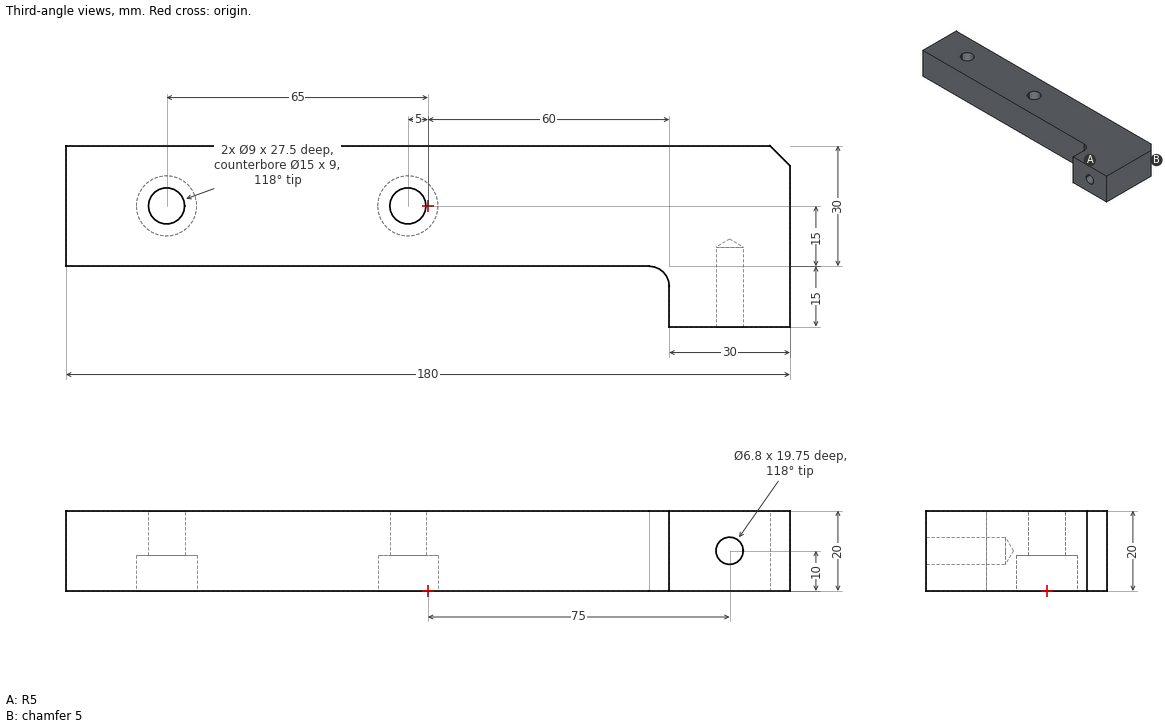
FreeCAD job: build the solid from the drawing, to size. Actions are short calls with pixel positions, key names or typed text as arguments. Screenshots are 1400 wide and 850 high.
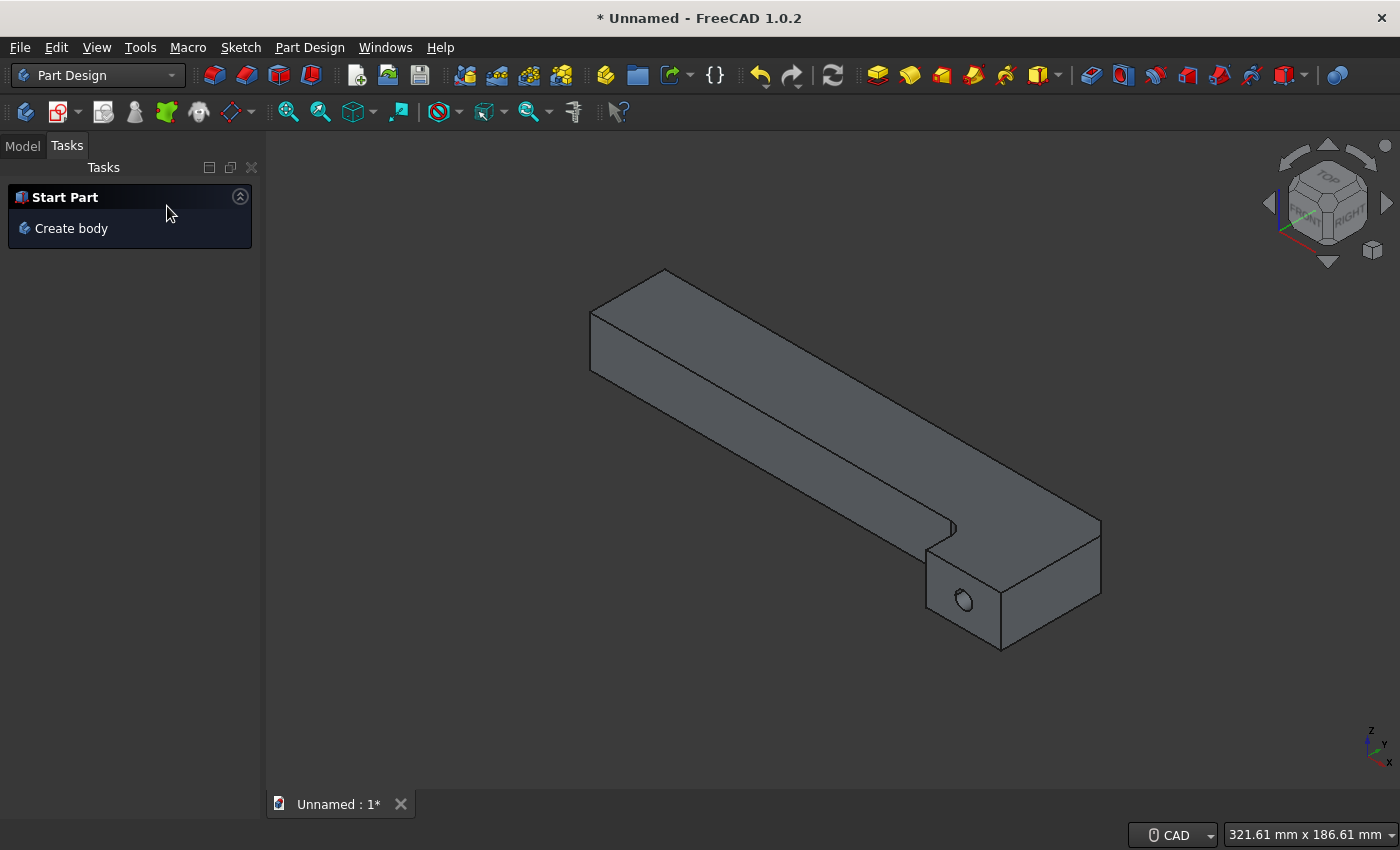
click(58, 112)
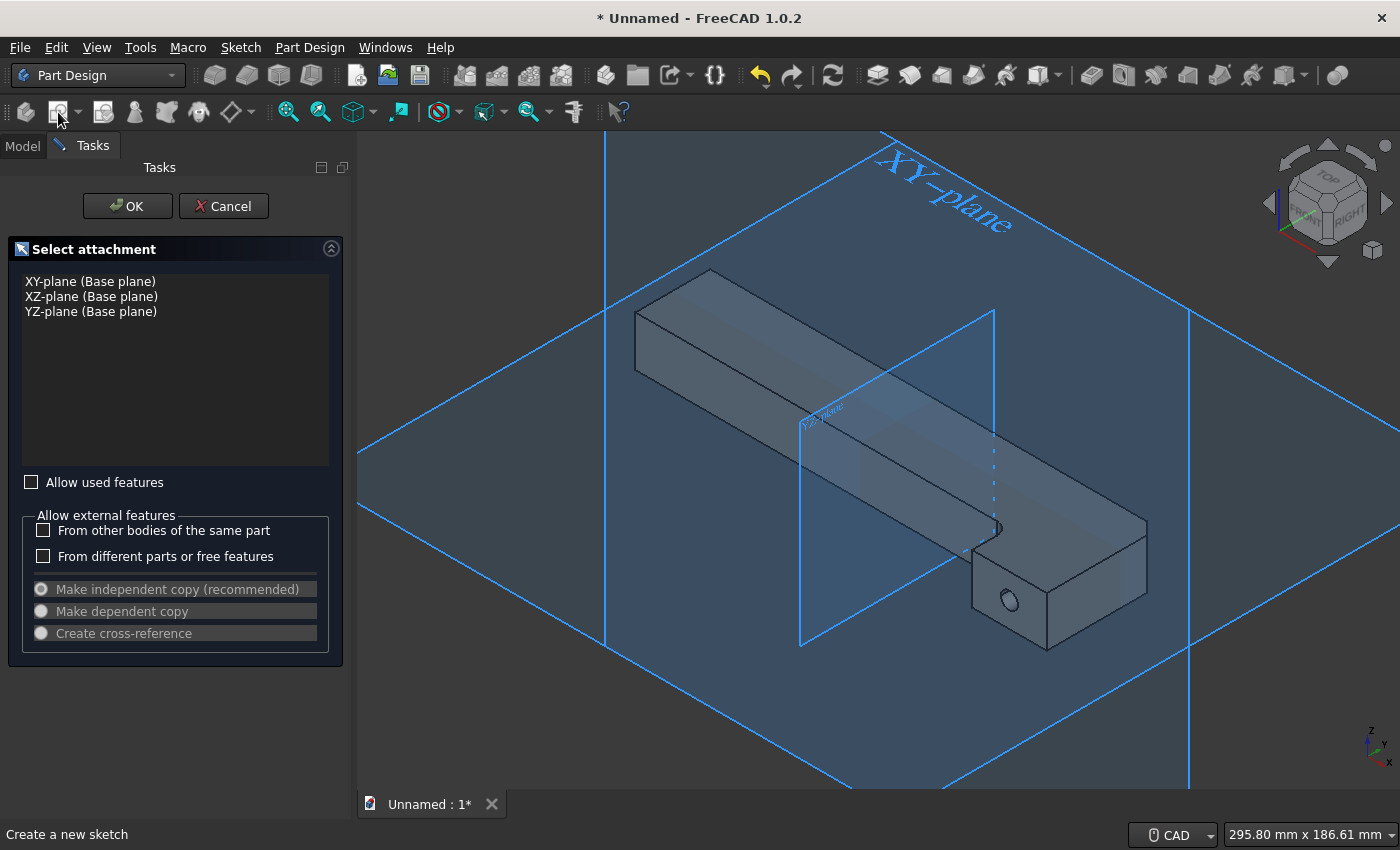
click(82, 282)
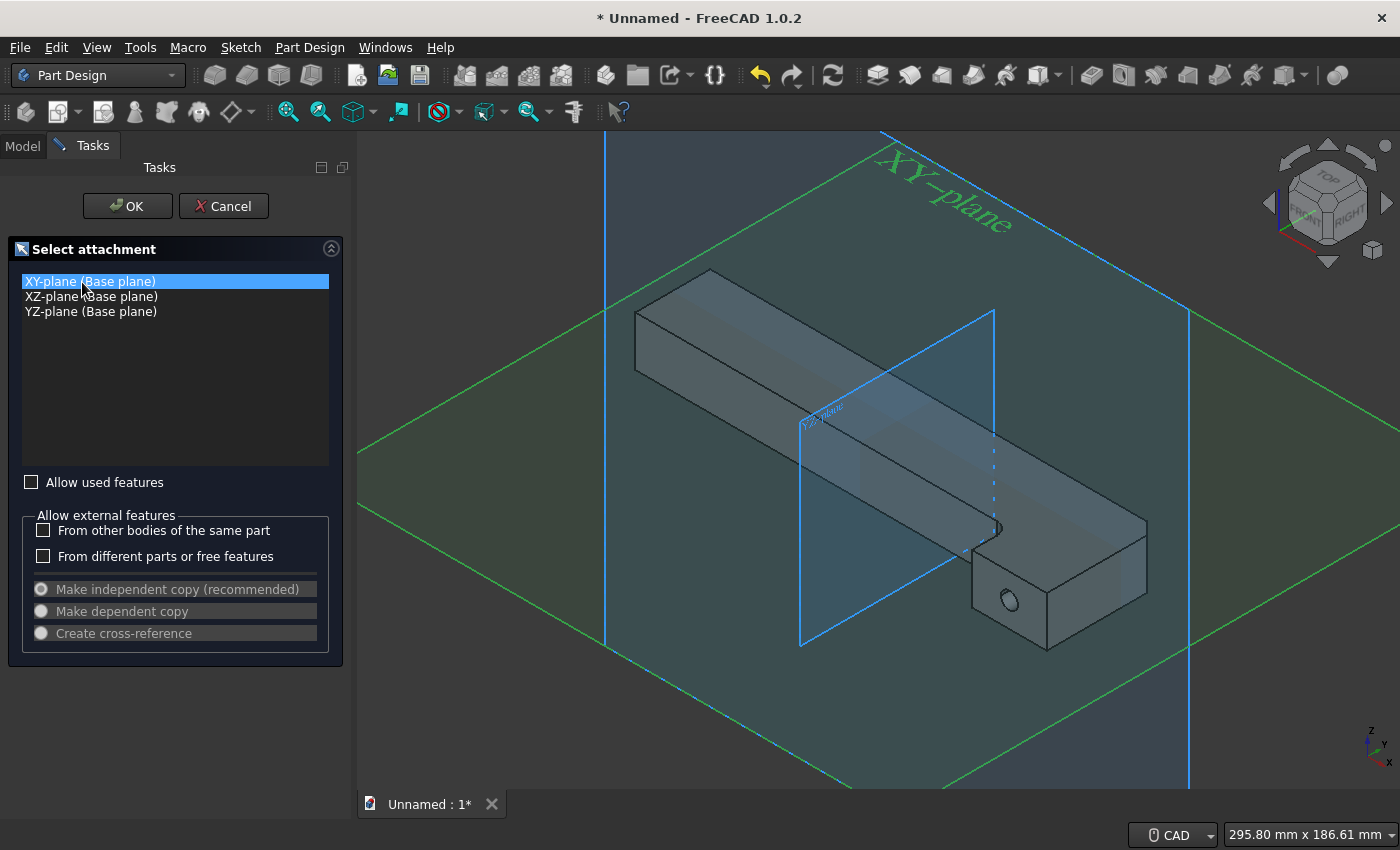
click(128, 206)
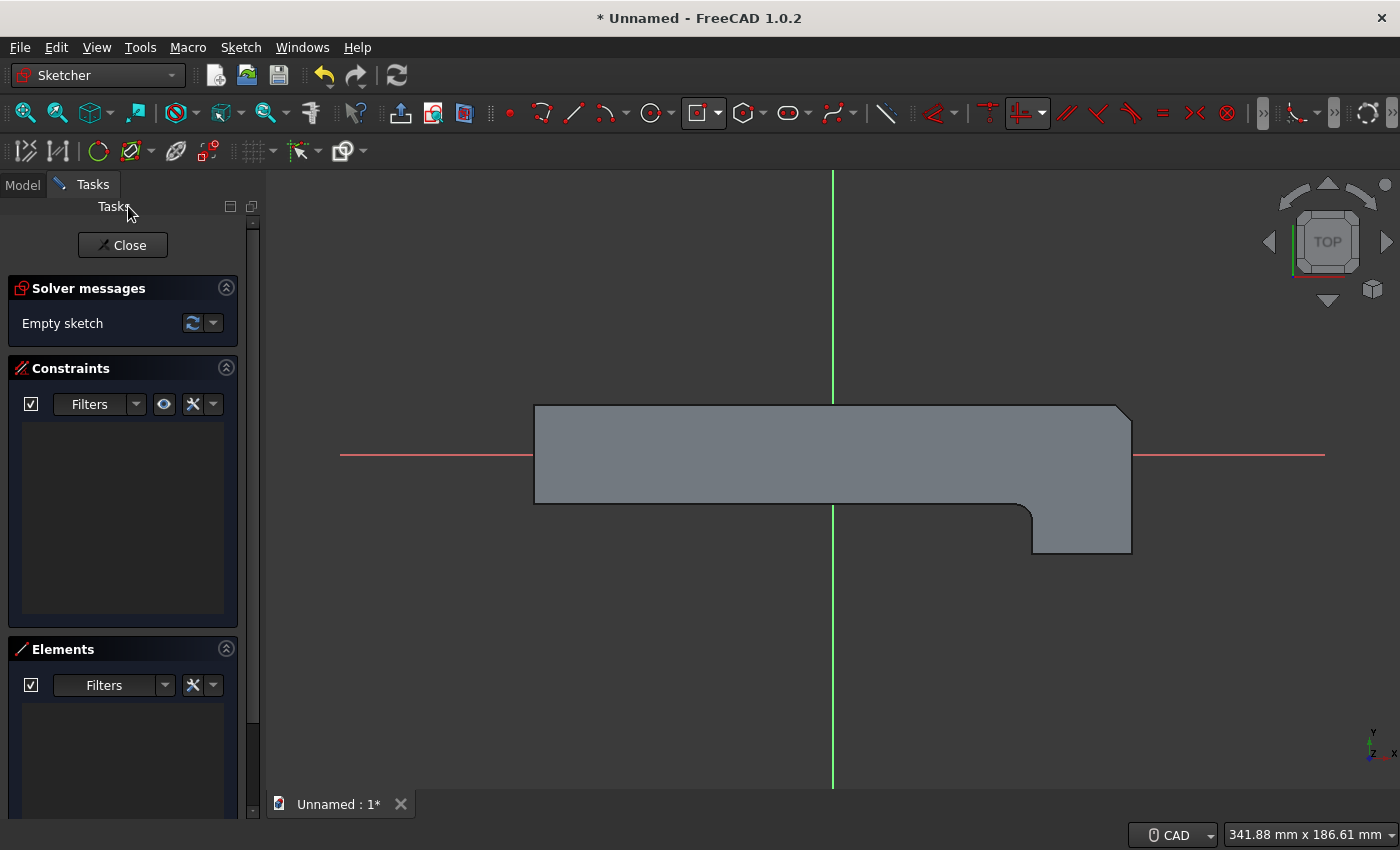
click(466, 114)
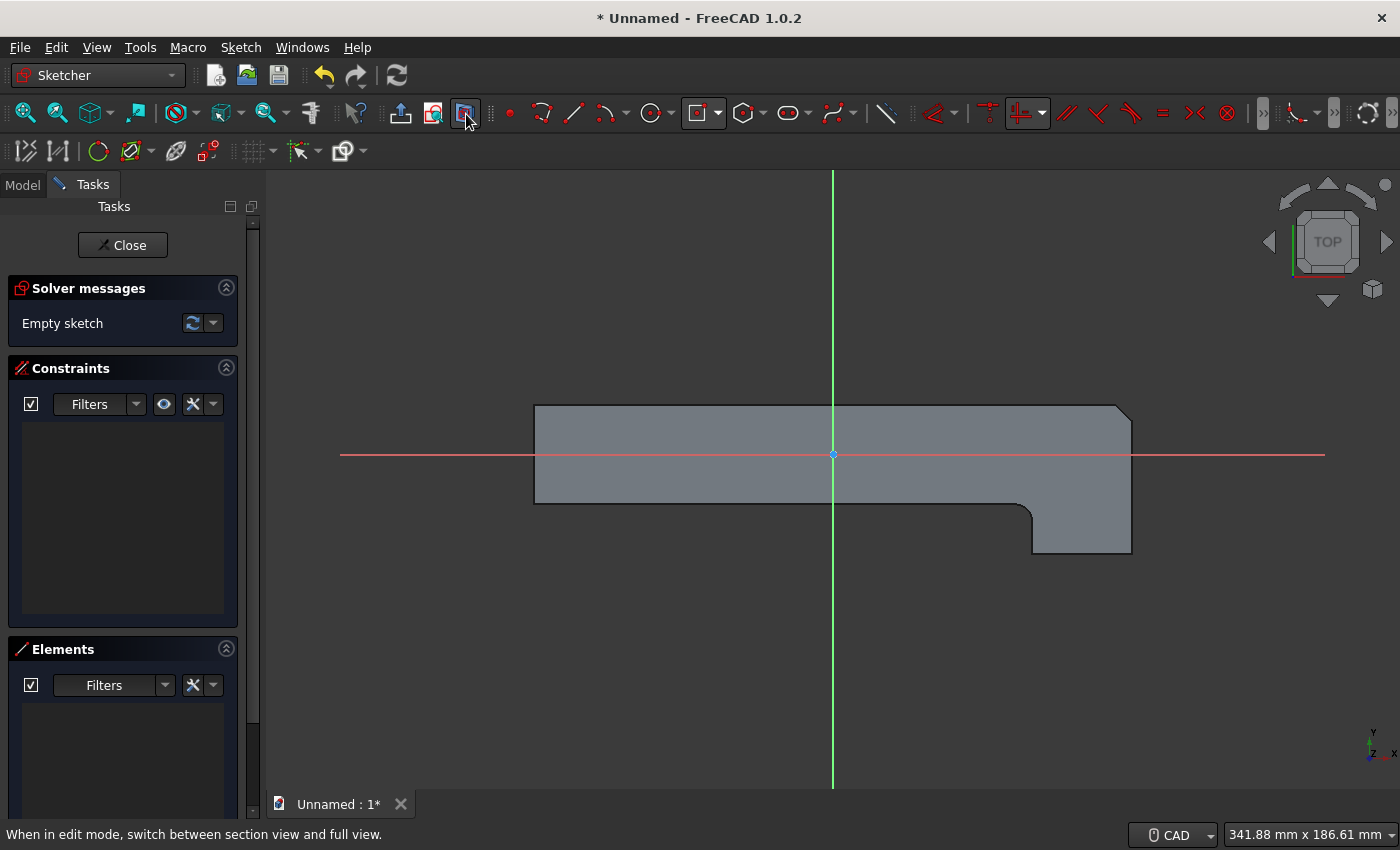
scroll(691, 440, up, 5)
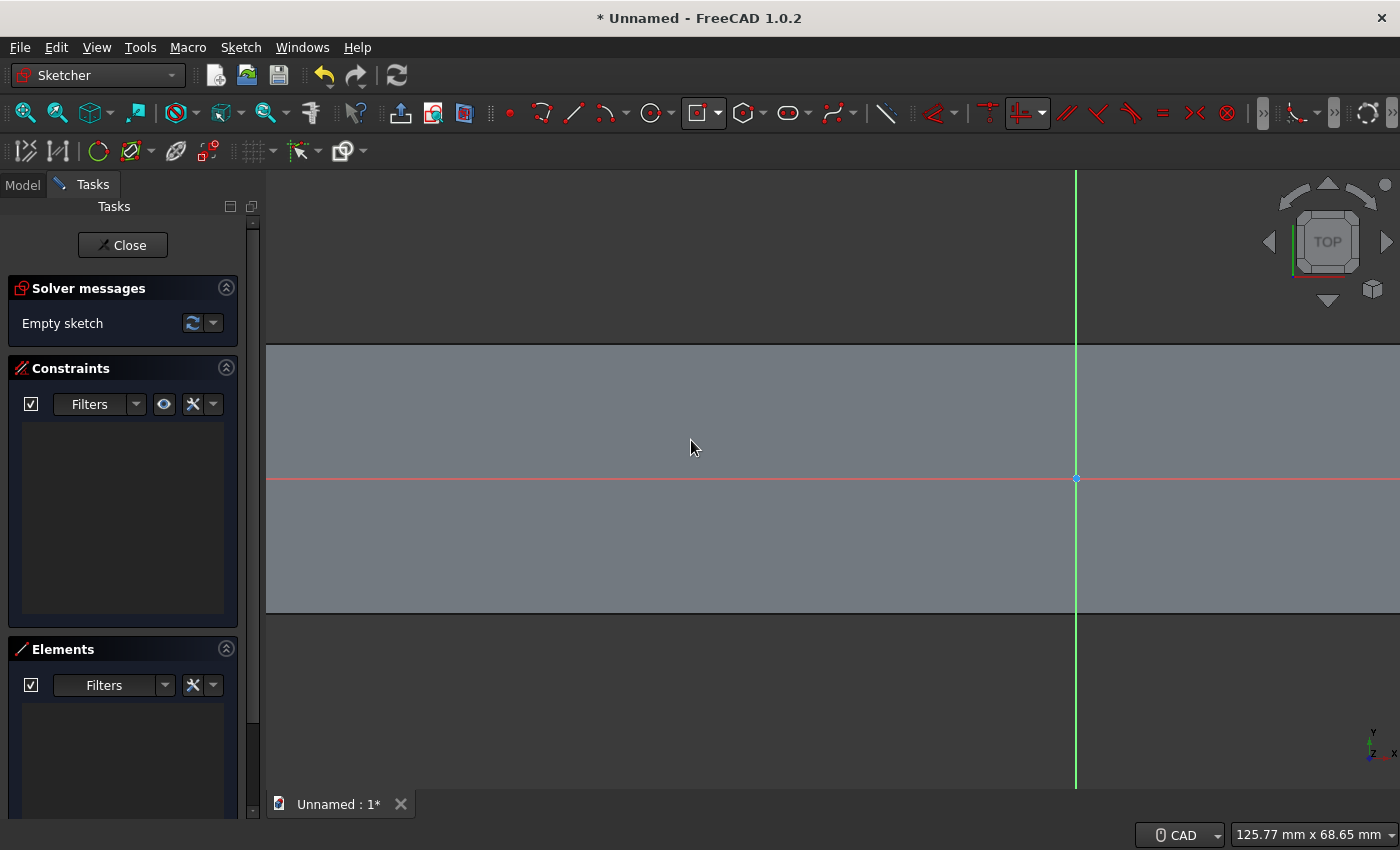
click(652, 114)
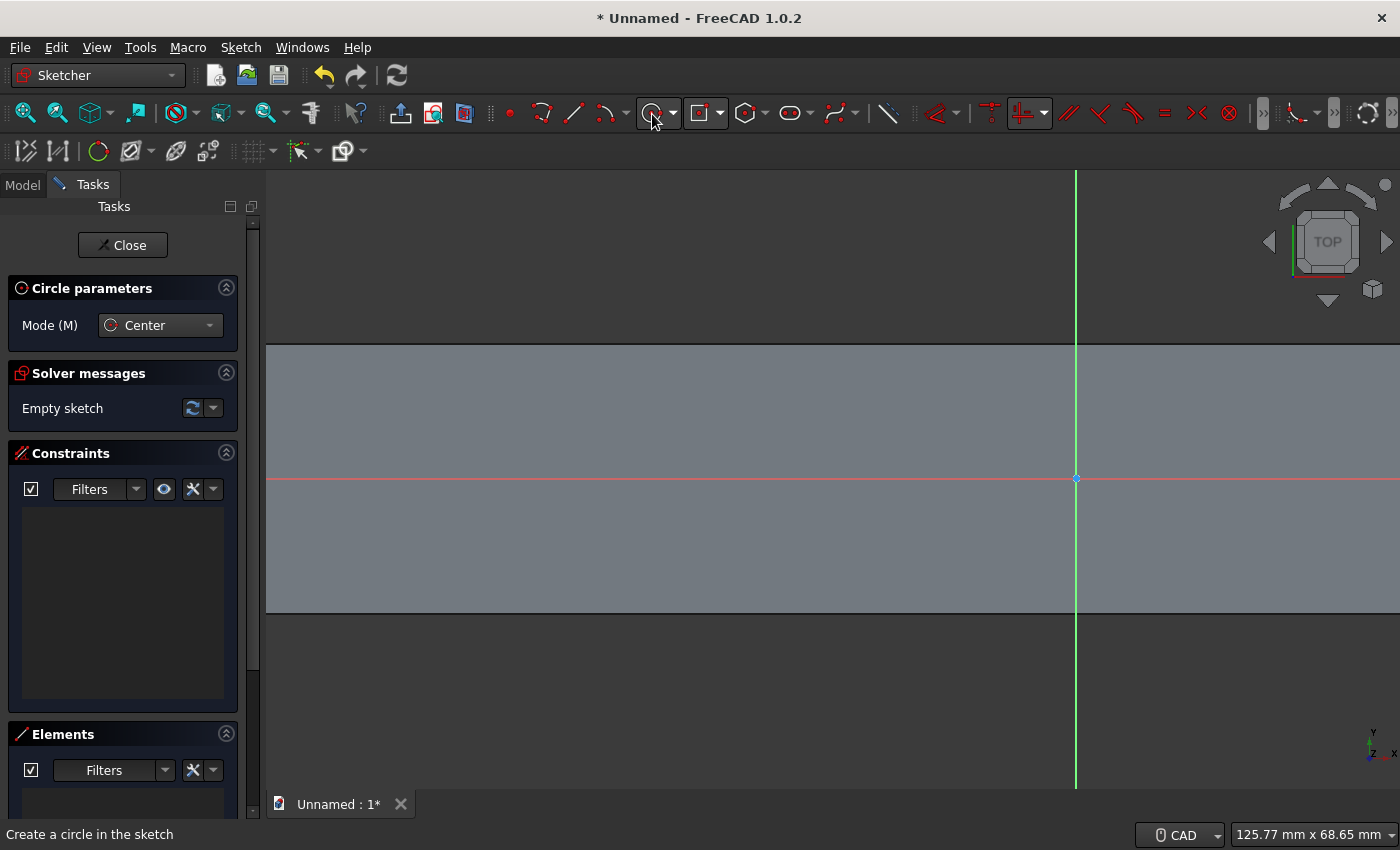
click(490, 479)
move(519, 450)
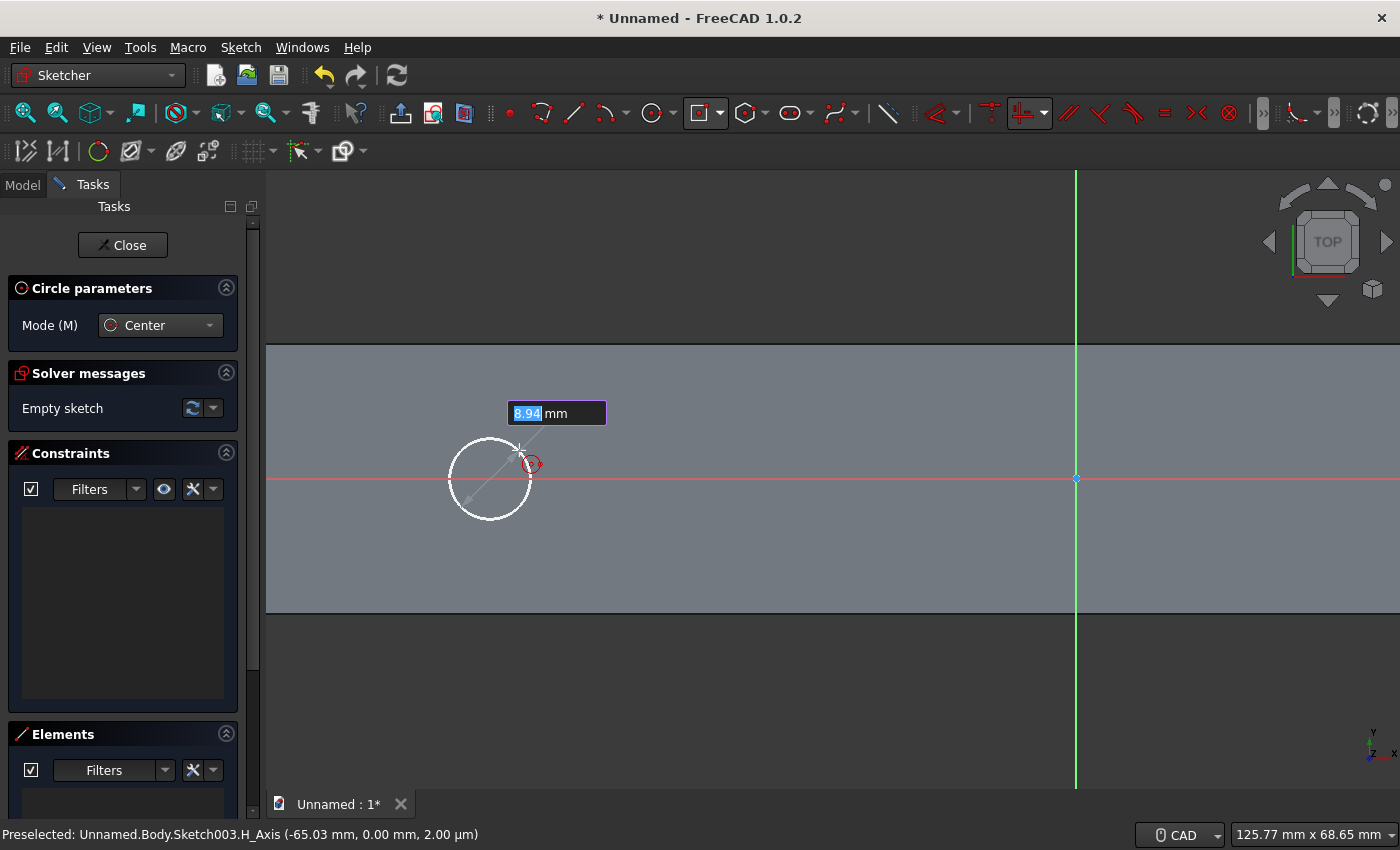
text(9)
key(Return)